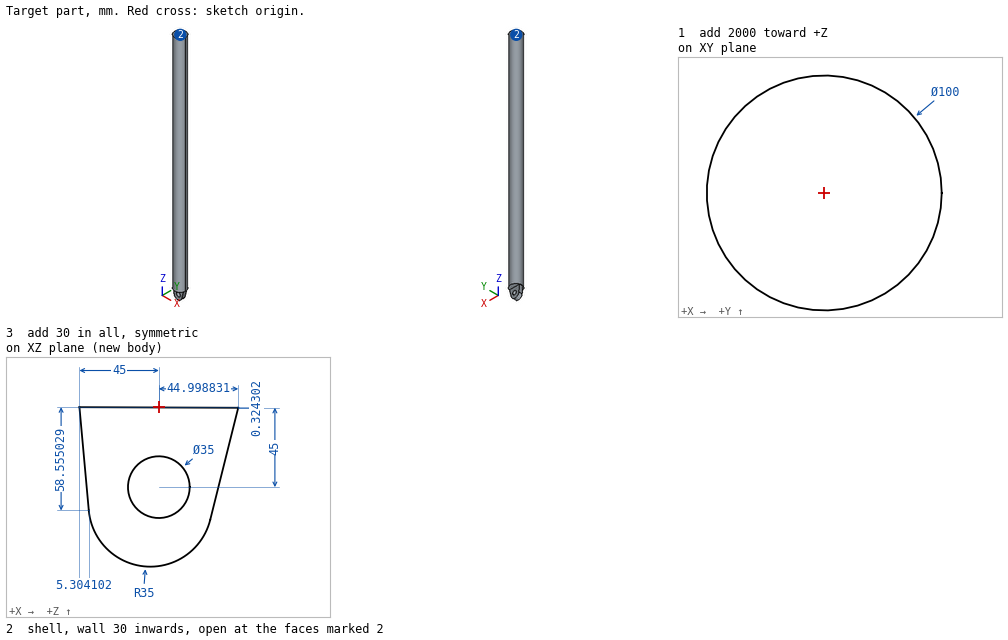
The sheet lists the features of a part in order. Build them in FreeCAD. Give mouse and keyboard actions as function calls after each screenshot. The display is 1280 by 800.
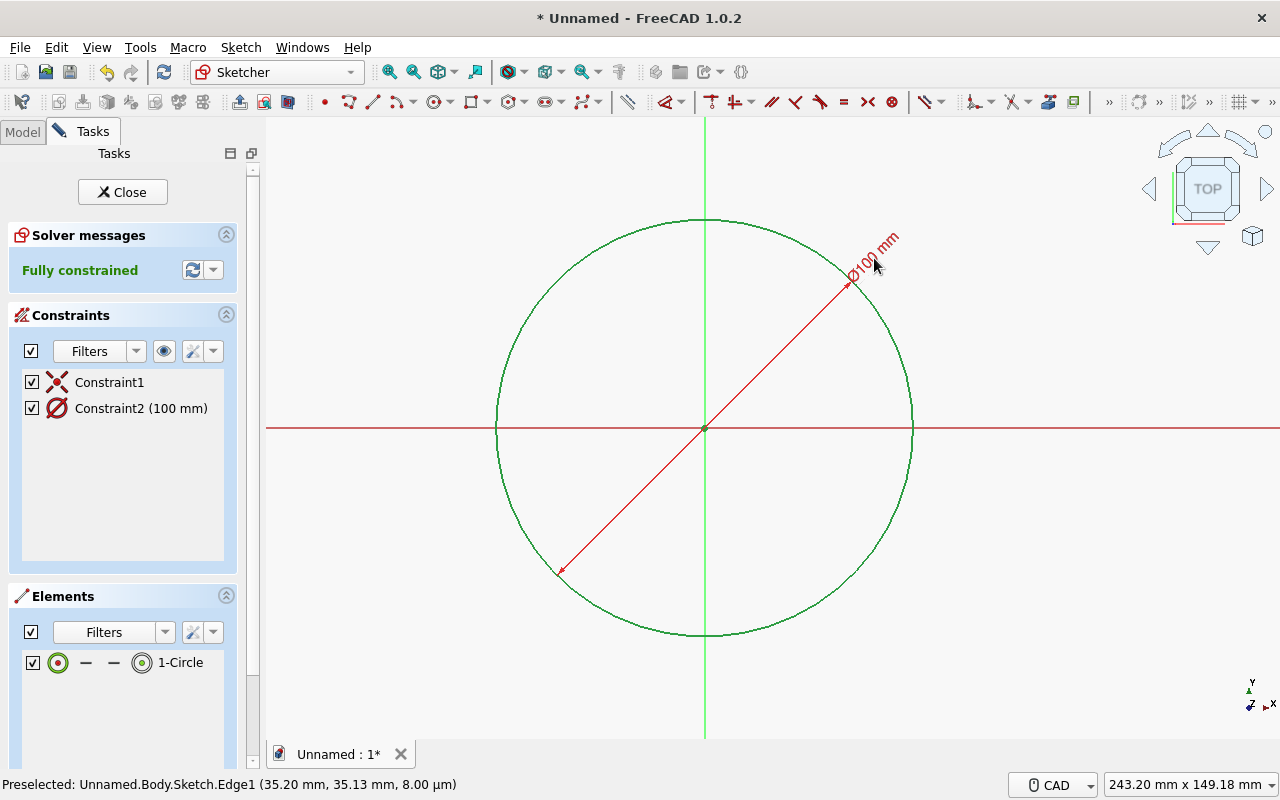
click(123, 192)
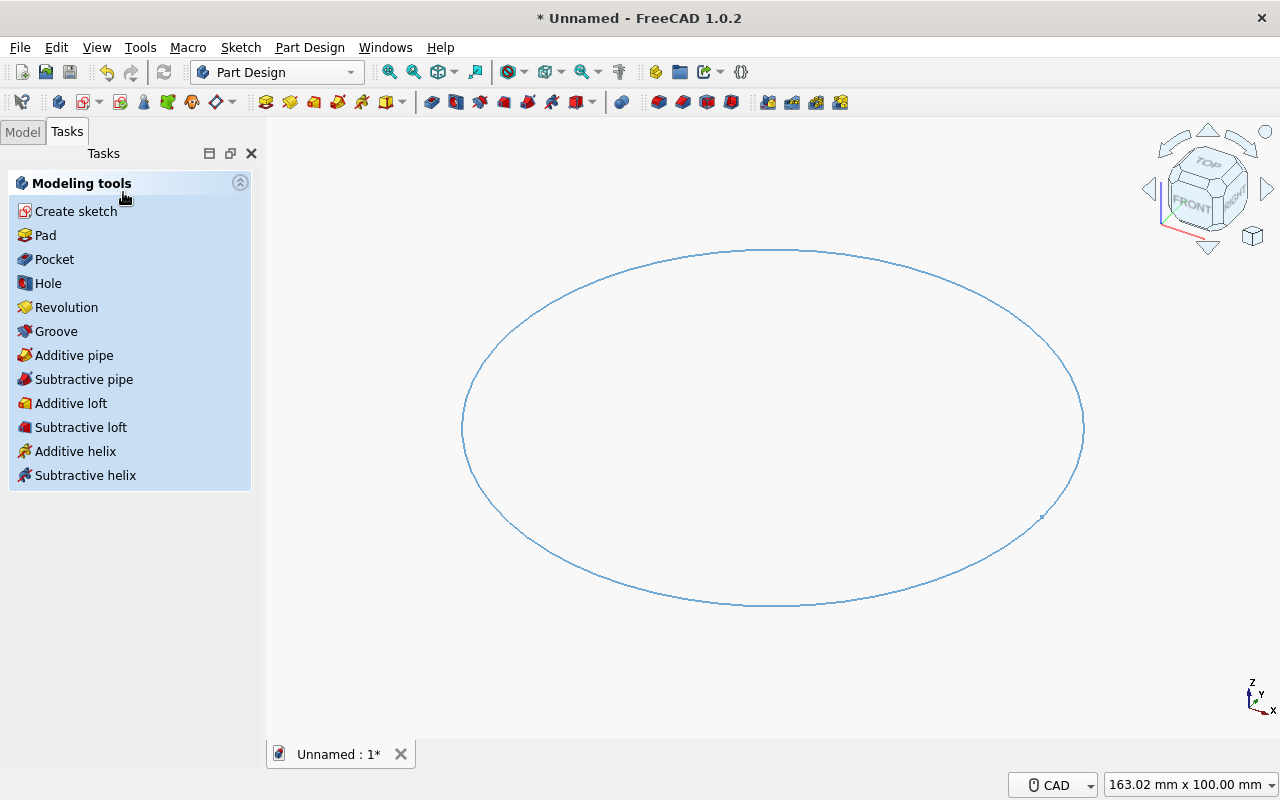
click(266, 102)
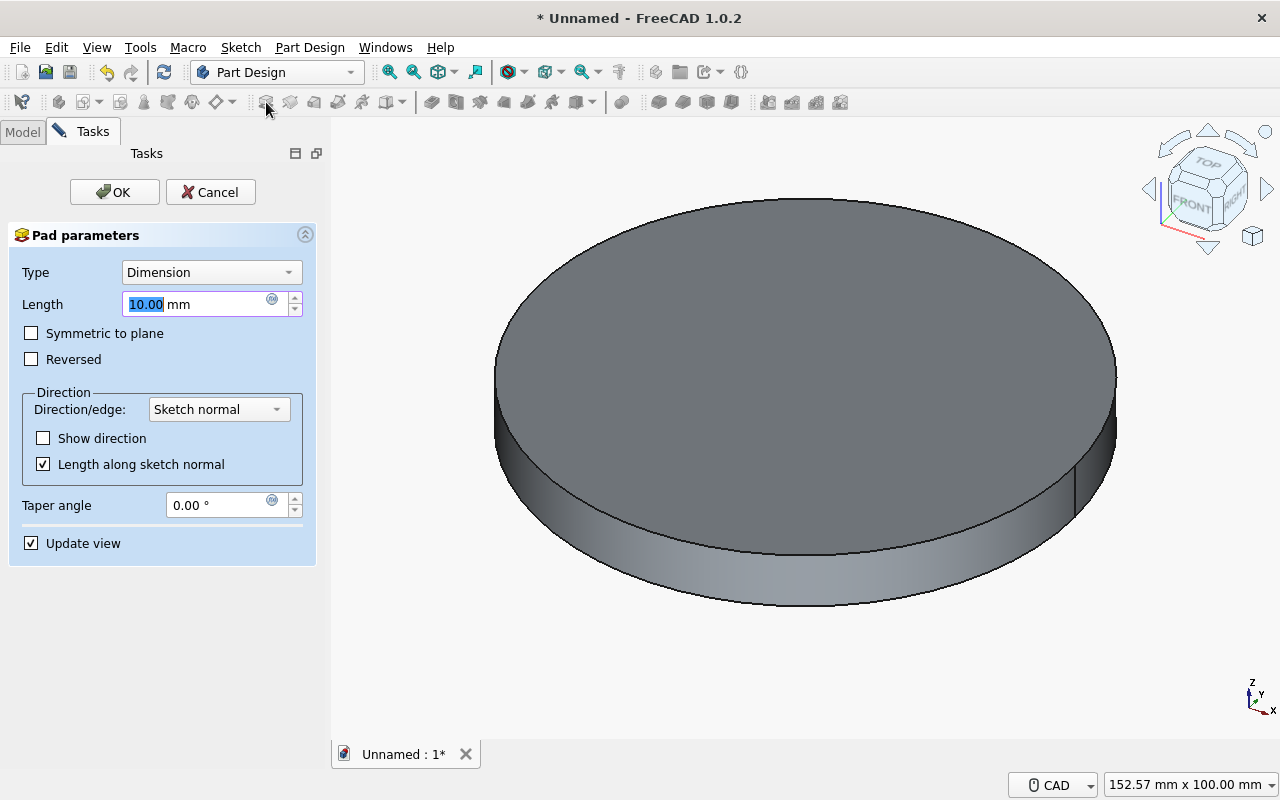
text(2000)
key(Tab)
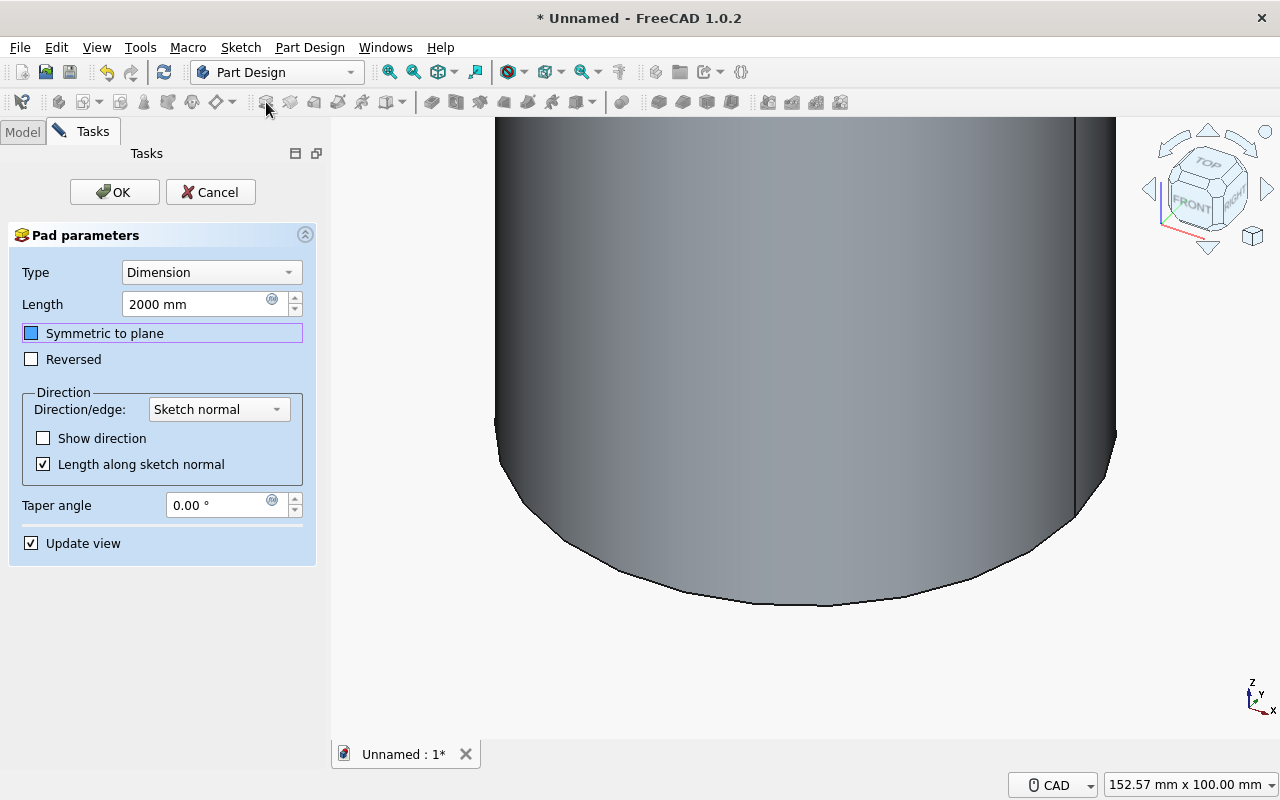
click(115, 192)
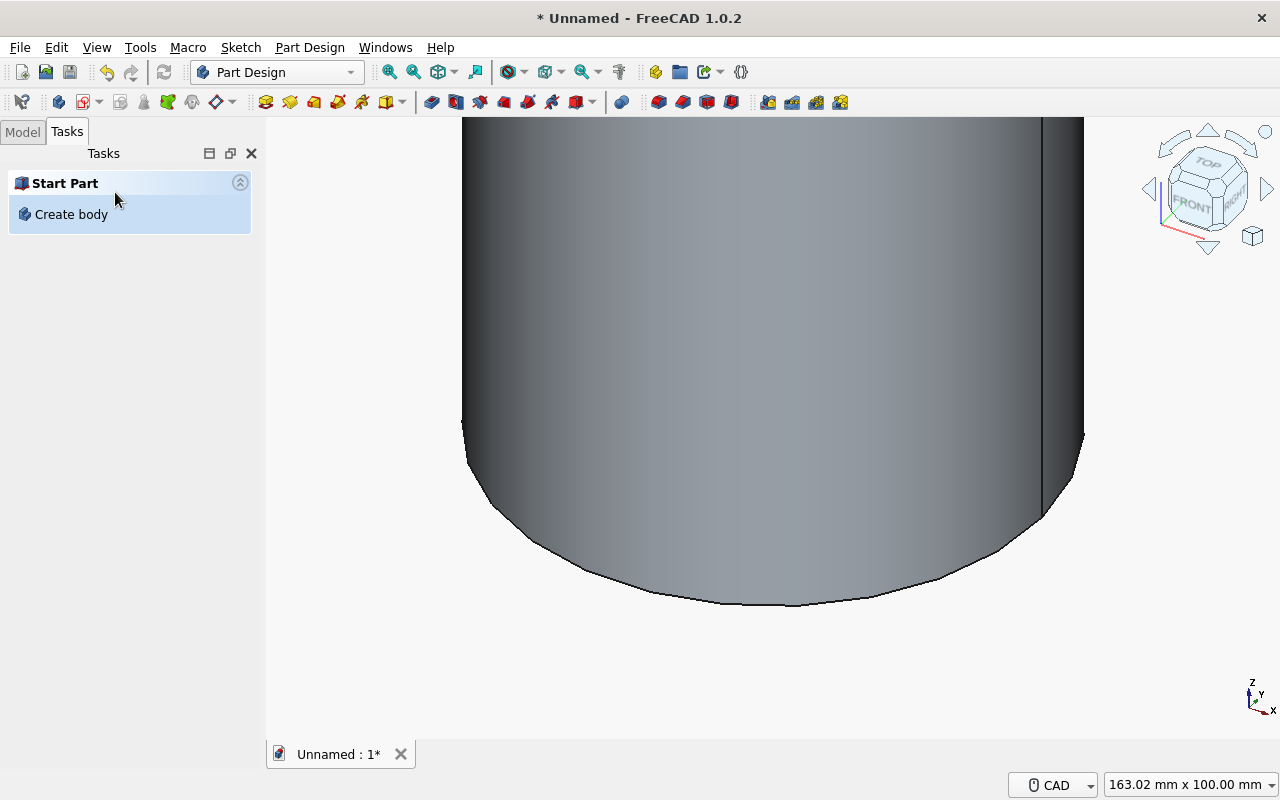
click(390, 72)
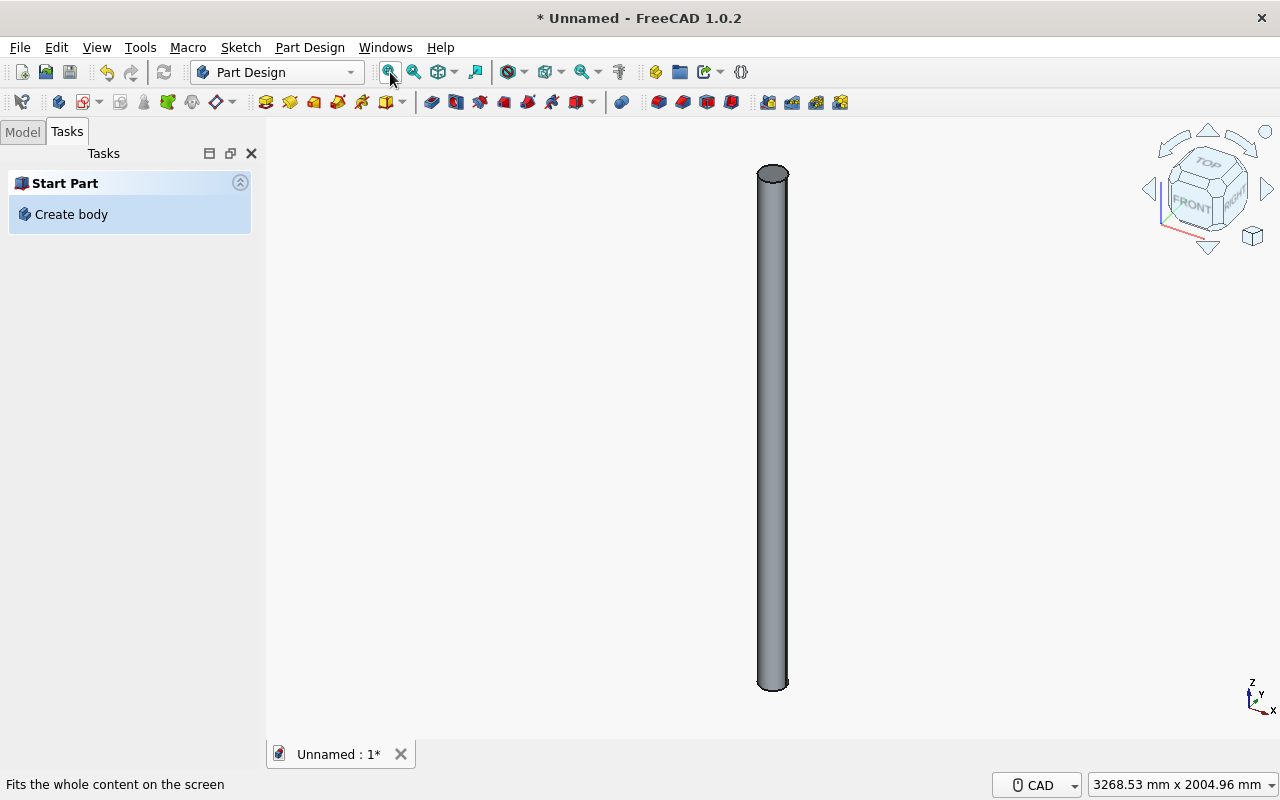
click(773, 173)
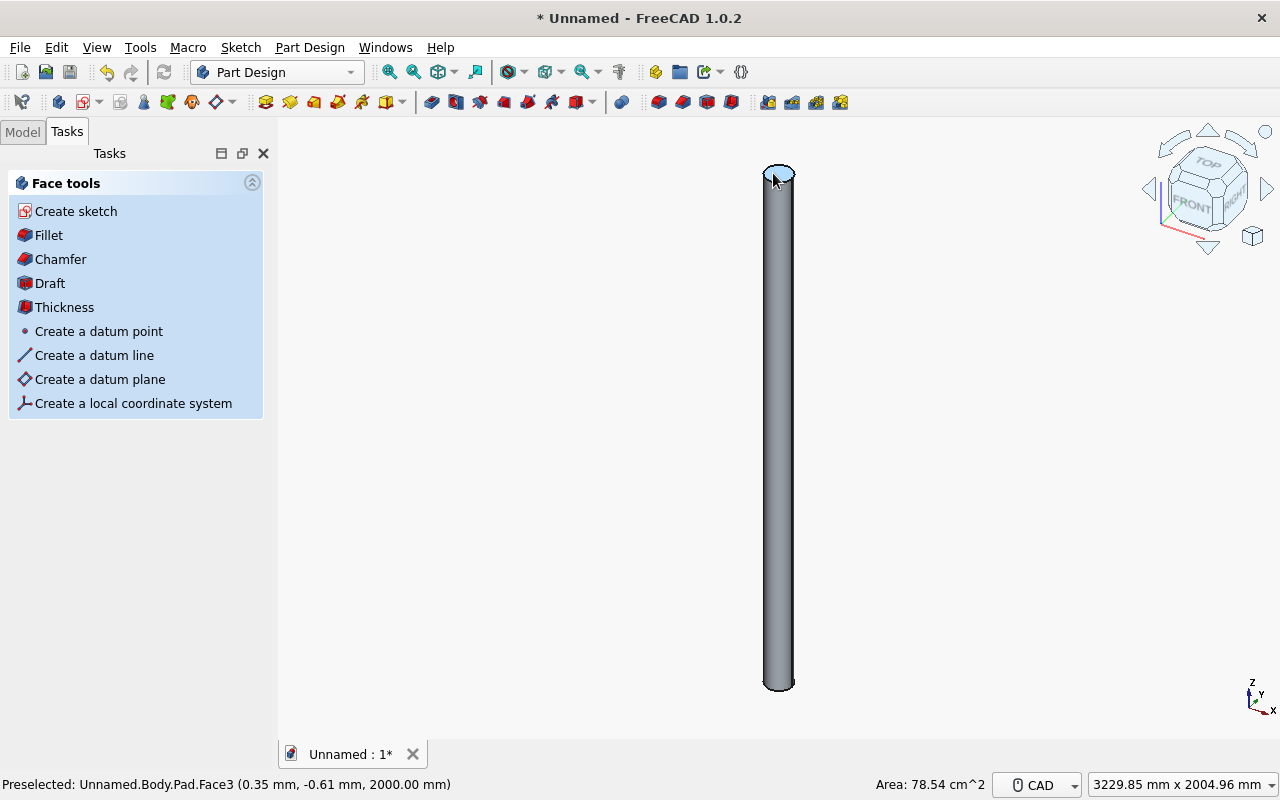
click(732, 102)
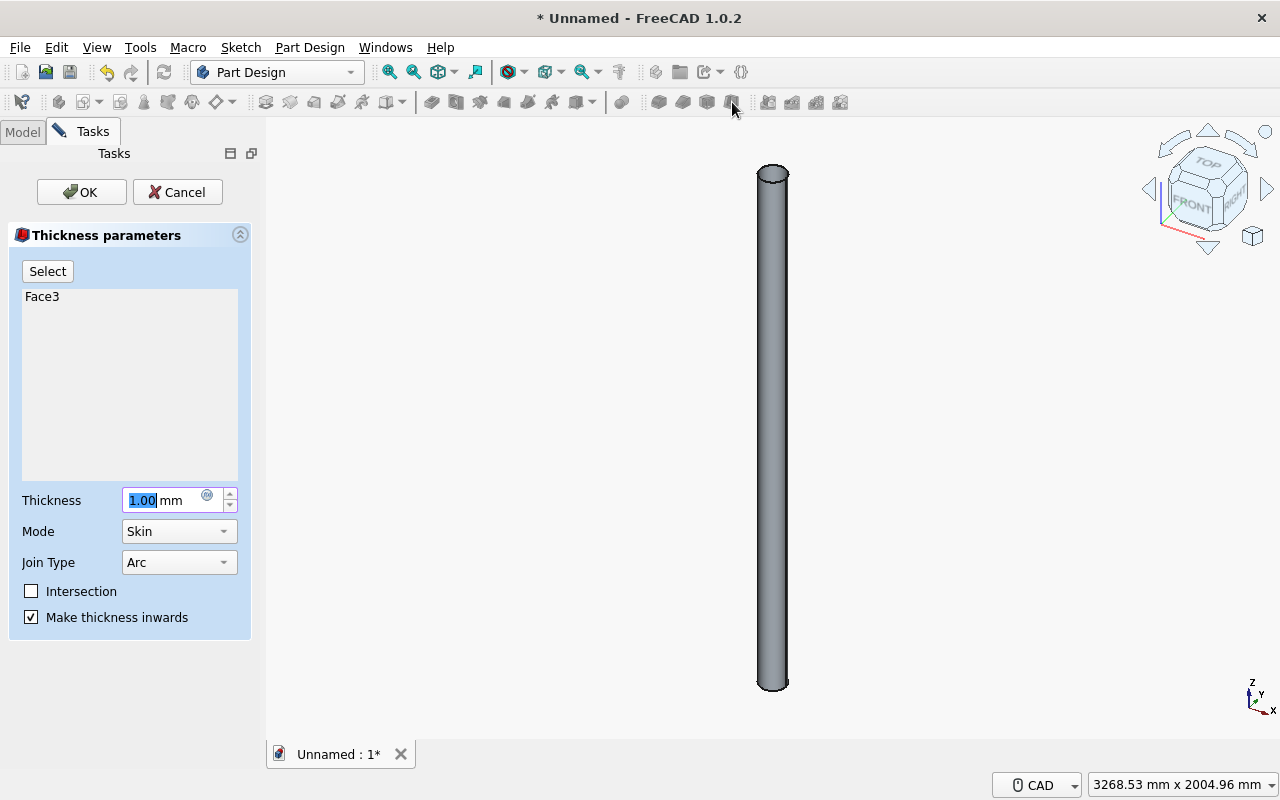
text(30)
key(Tab)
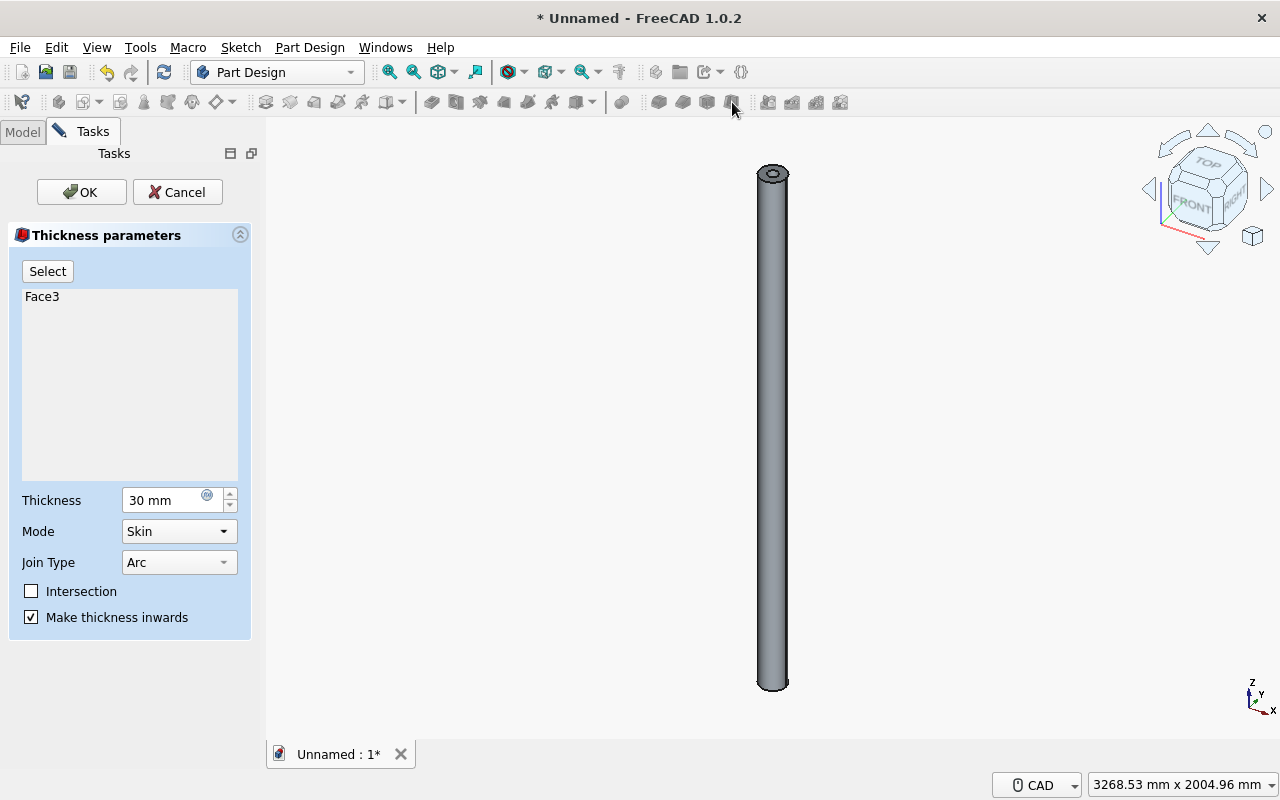
click(180, 562)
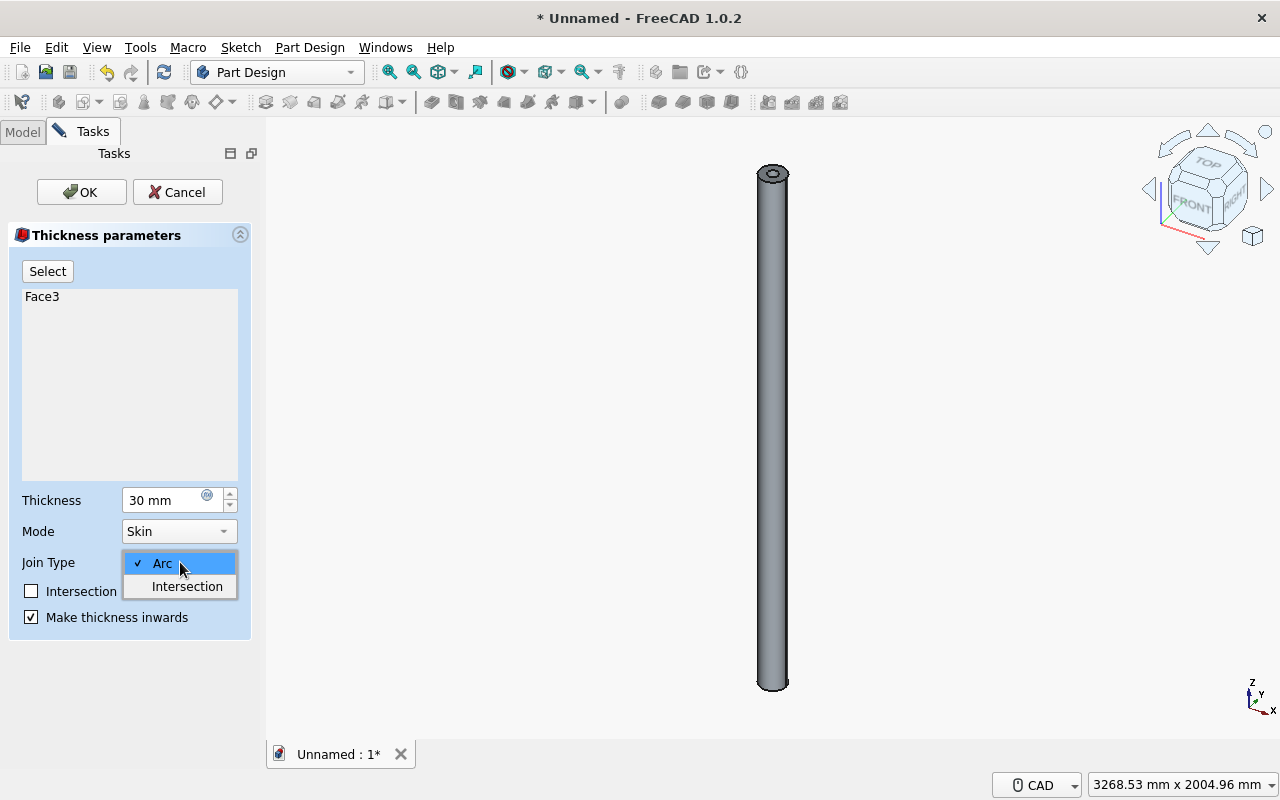
click(179, 586)